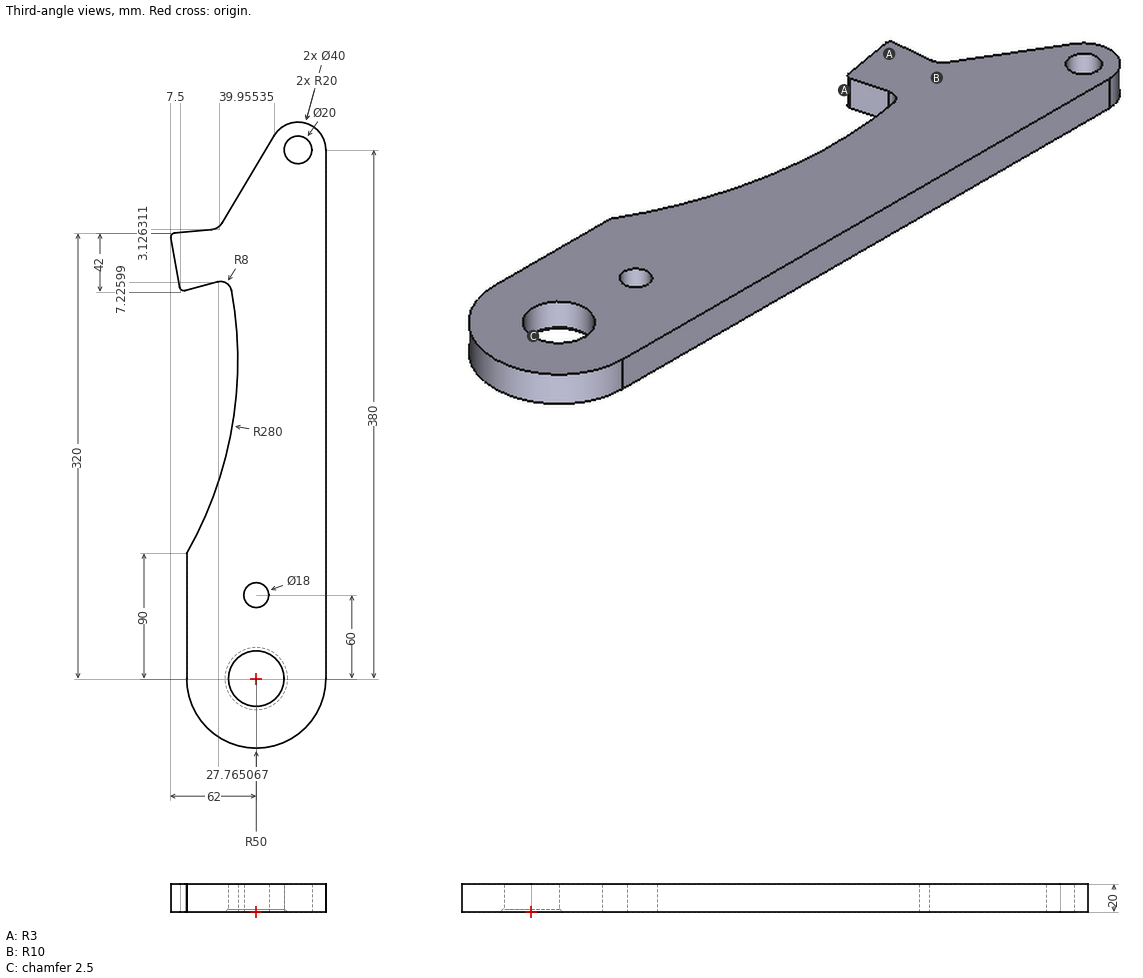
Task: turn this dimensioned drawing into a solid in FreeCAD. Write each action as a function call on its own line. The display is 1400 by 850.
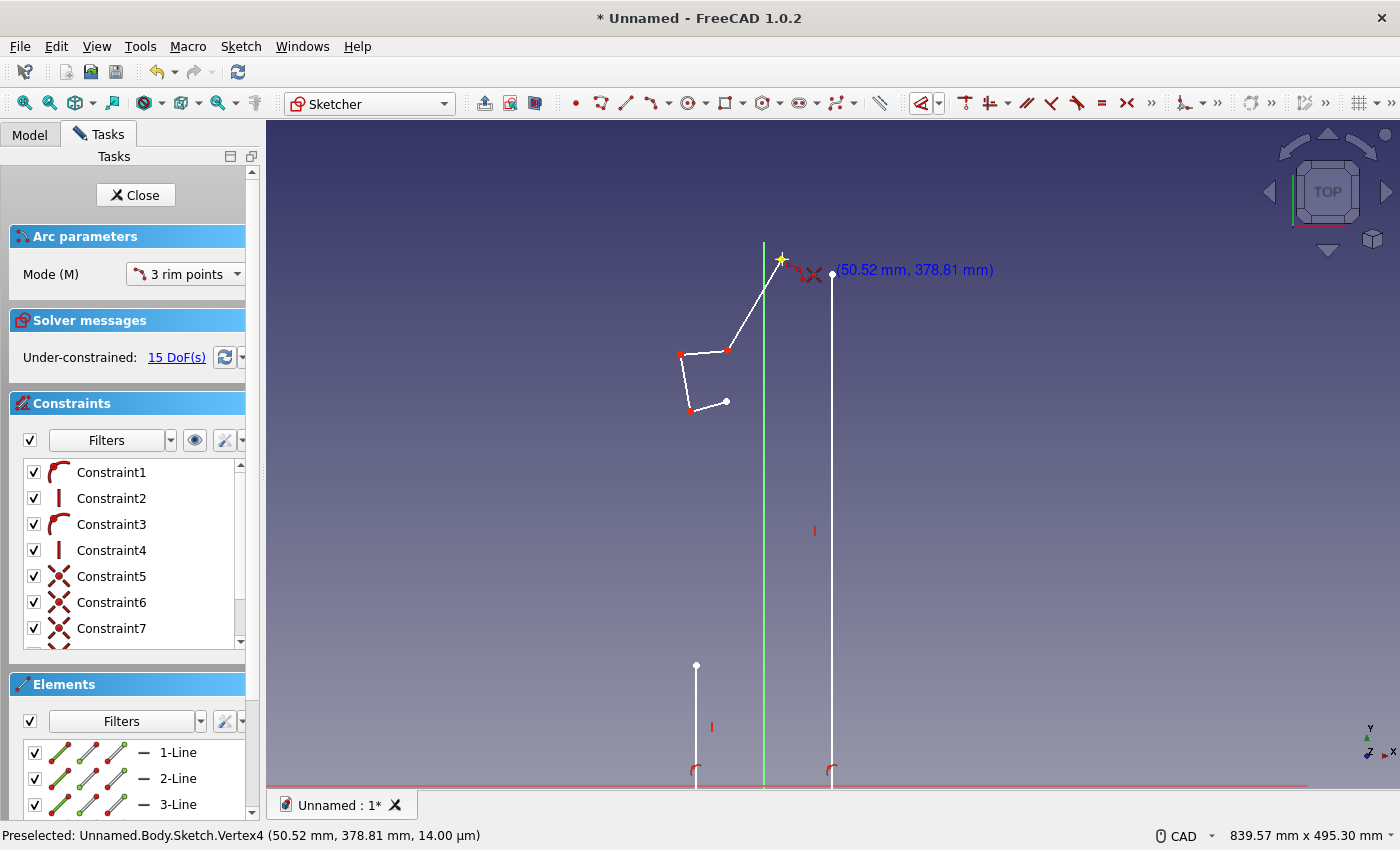
click(782, 260)
click(811, 247)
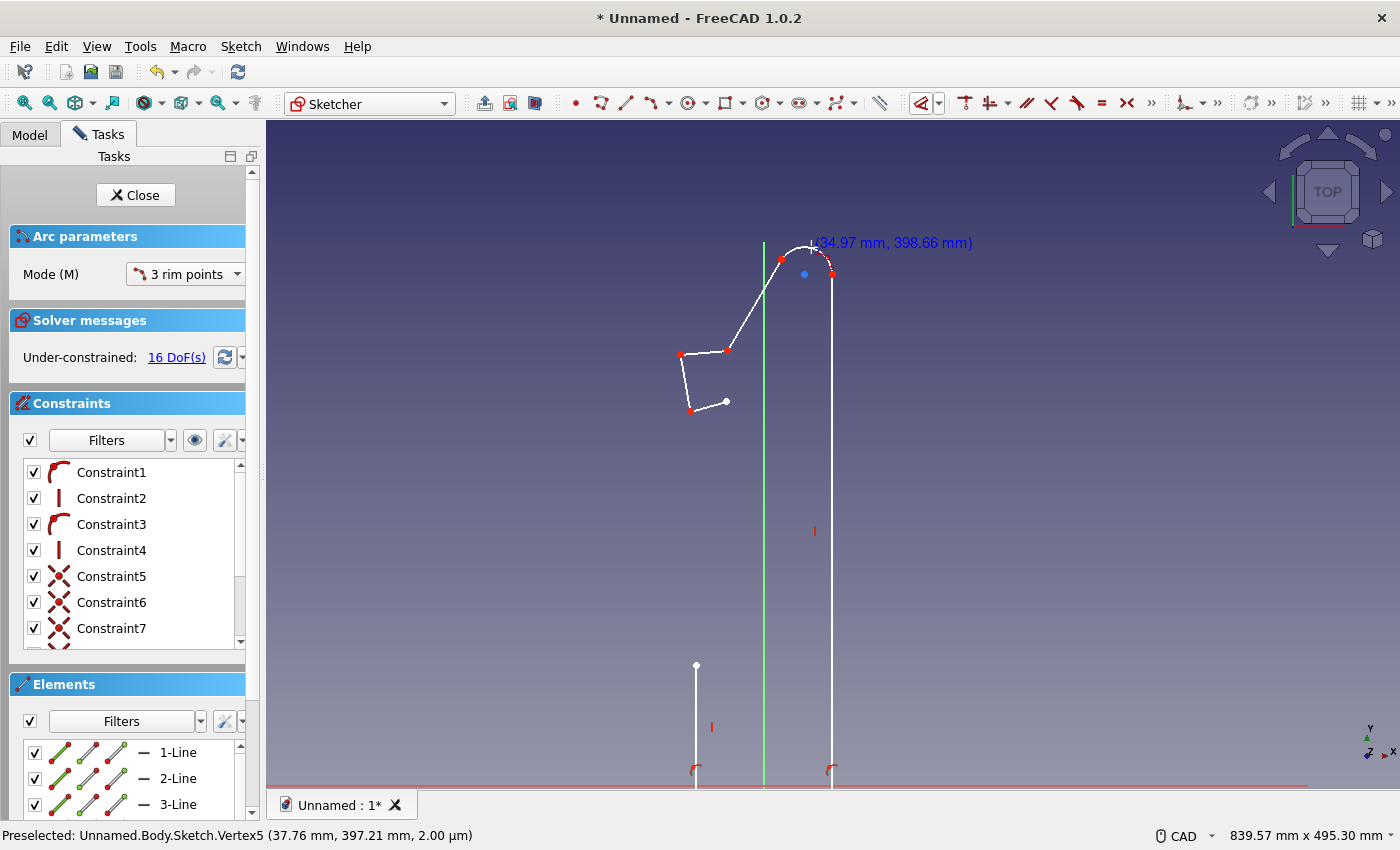
click(727, 402)
click(740, 410)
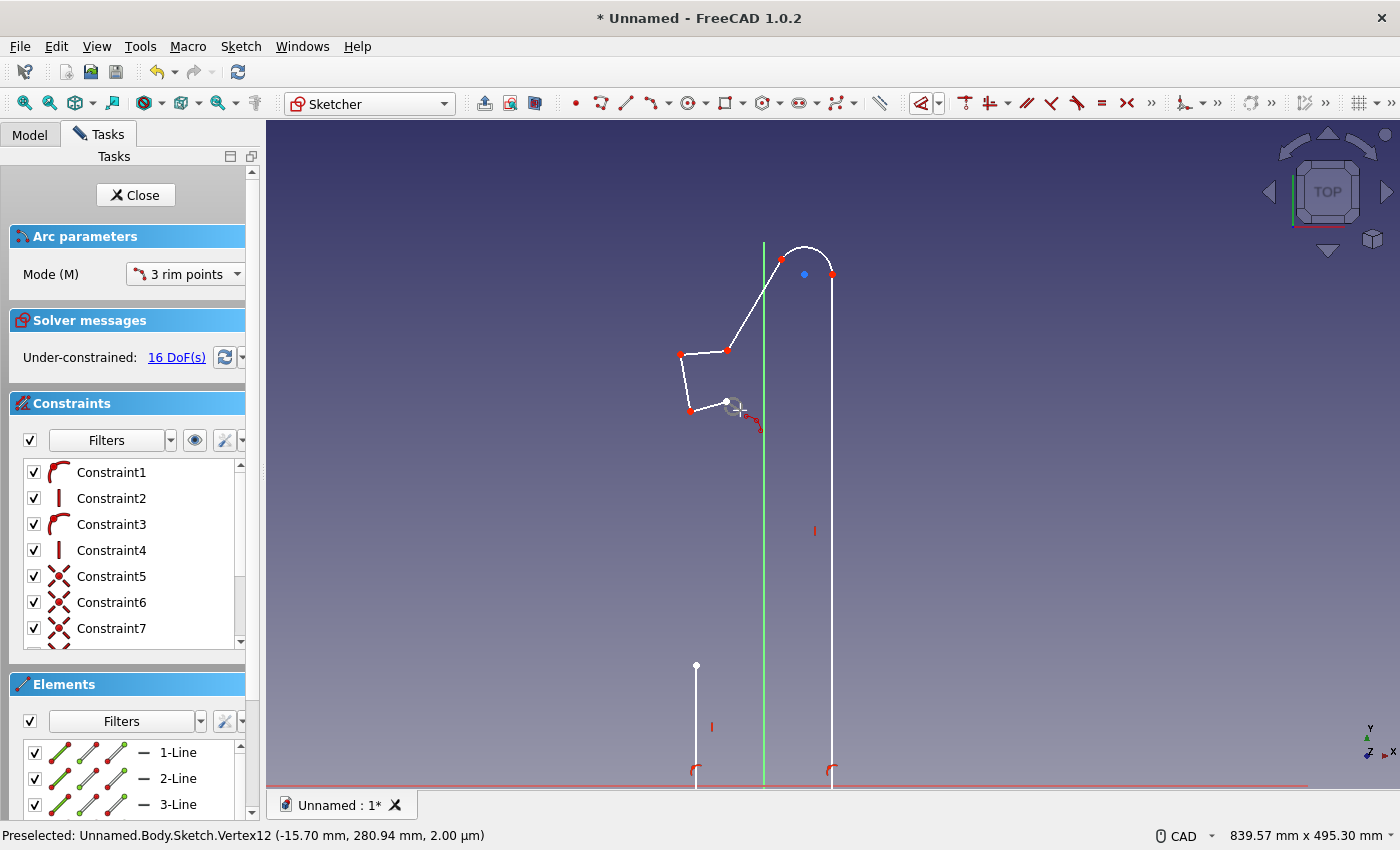
scroll(735, 403, up, 8)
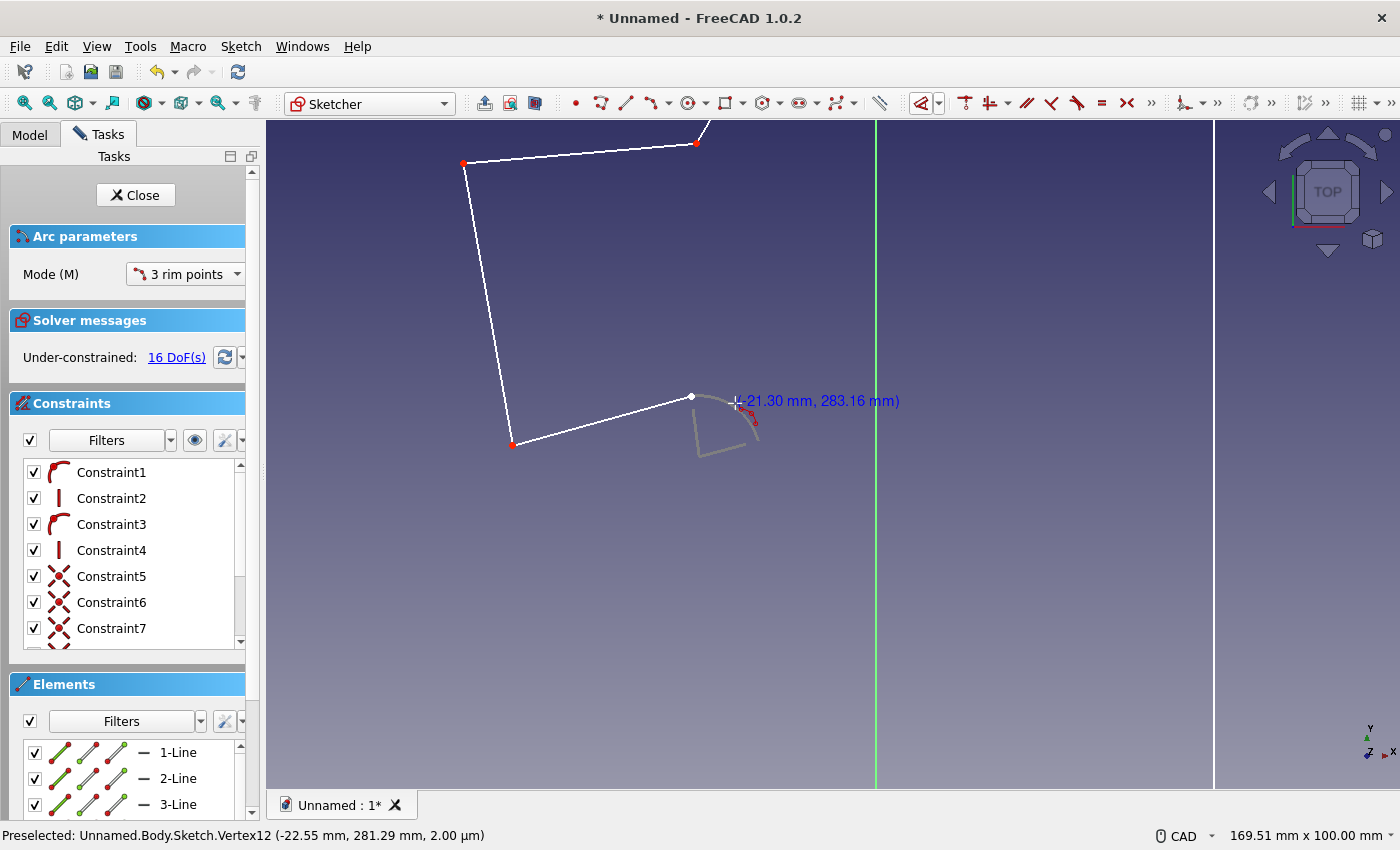
click(733, 399)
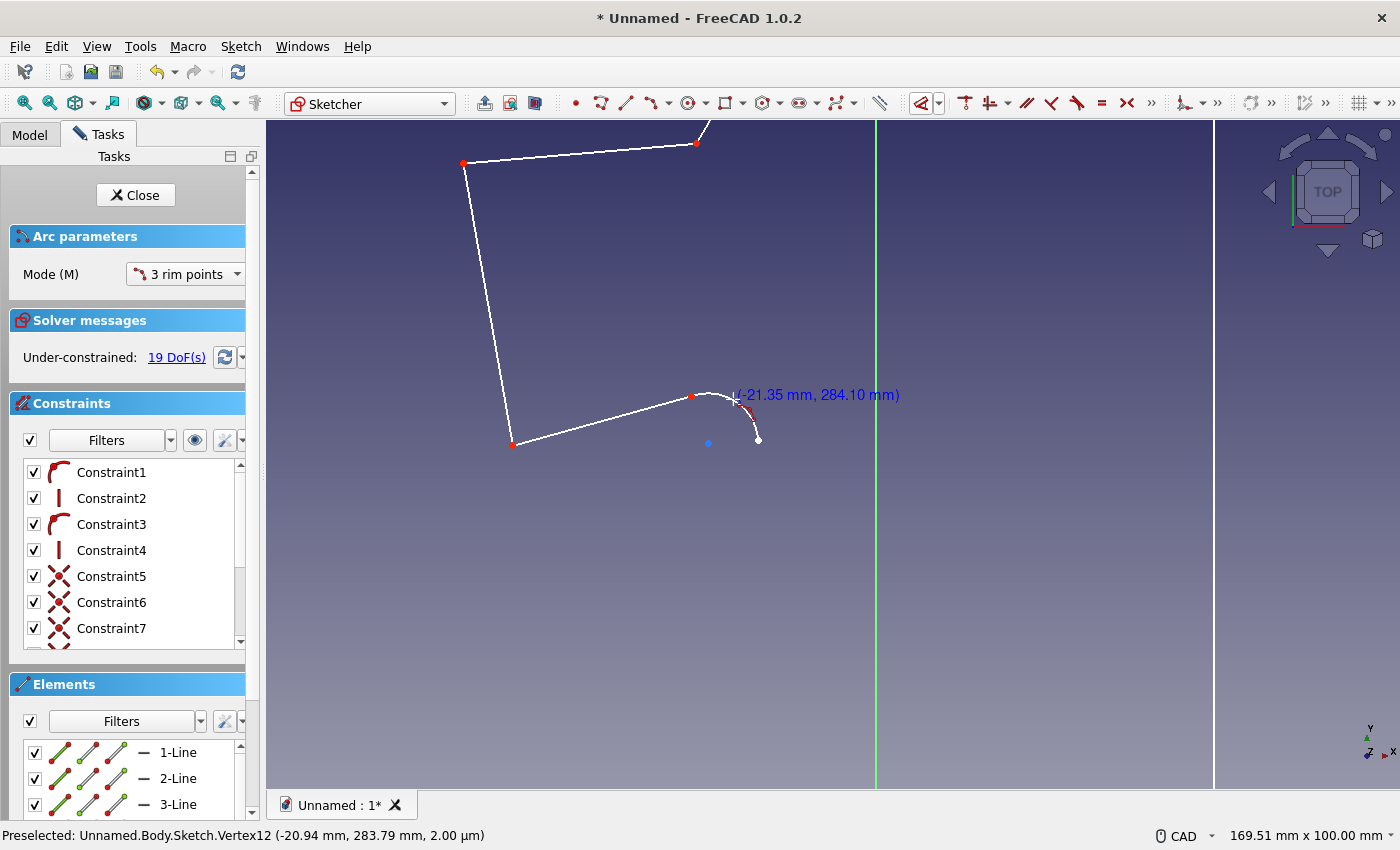
scroll(753, 348, down, 10)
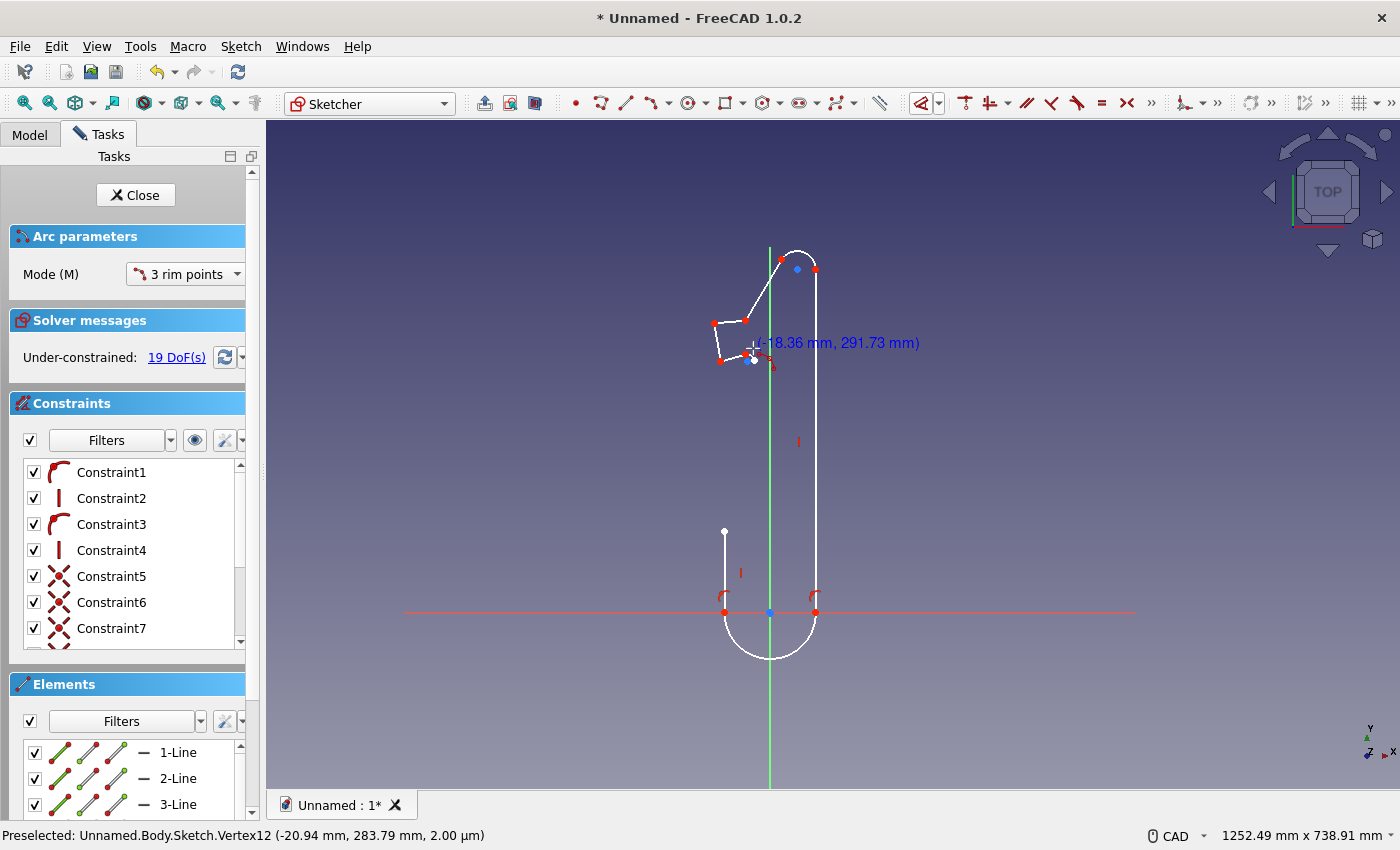
scroll(754, 360, up, 4)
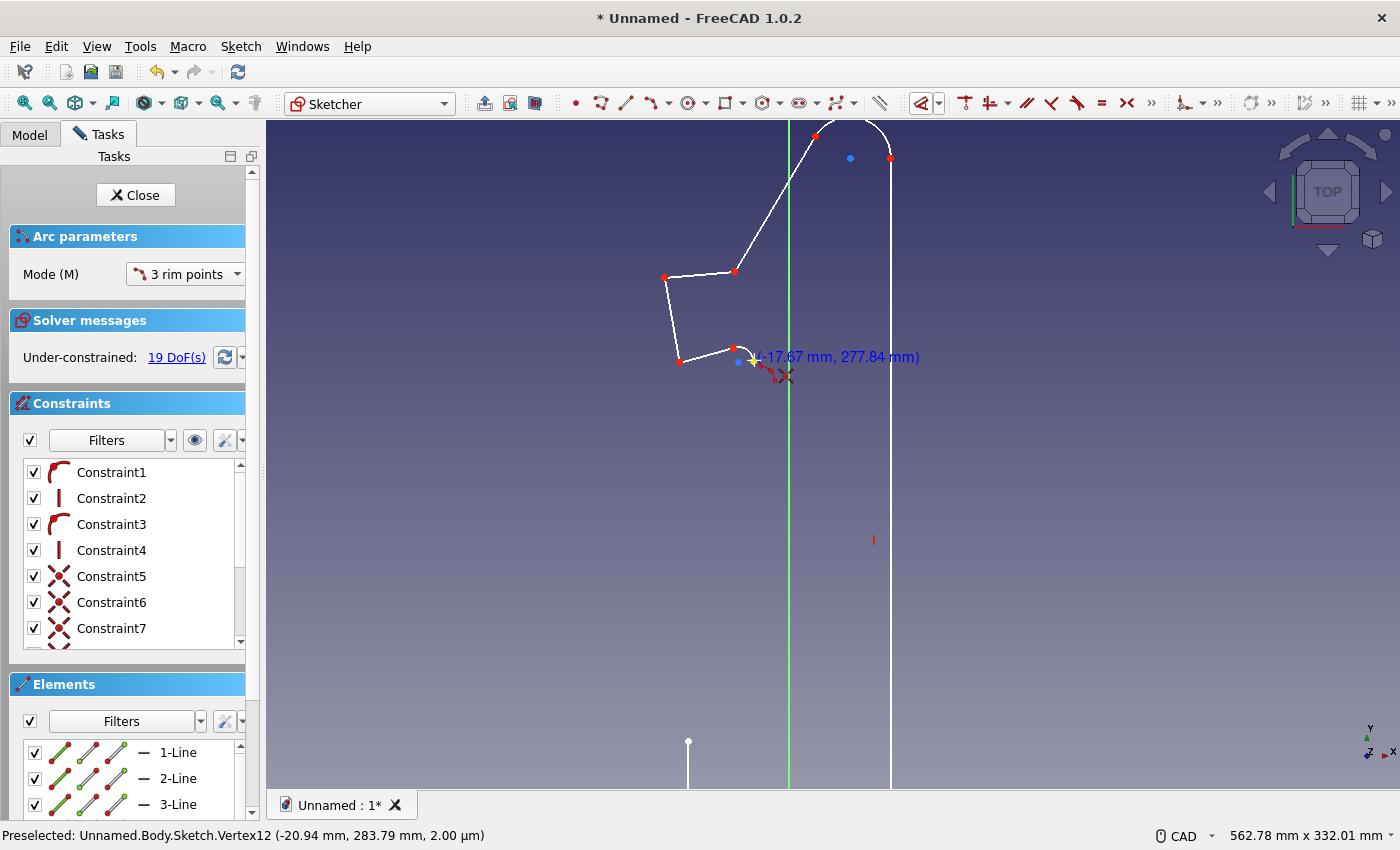
click(754, 362)
click(688, 741)
click(754, 556)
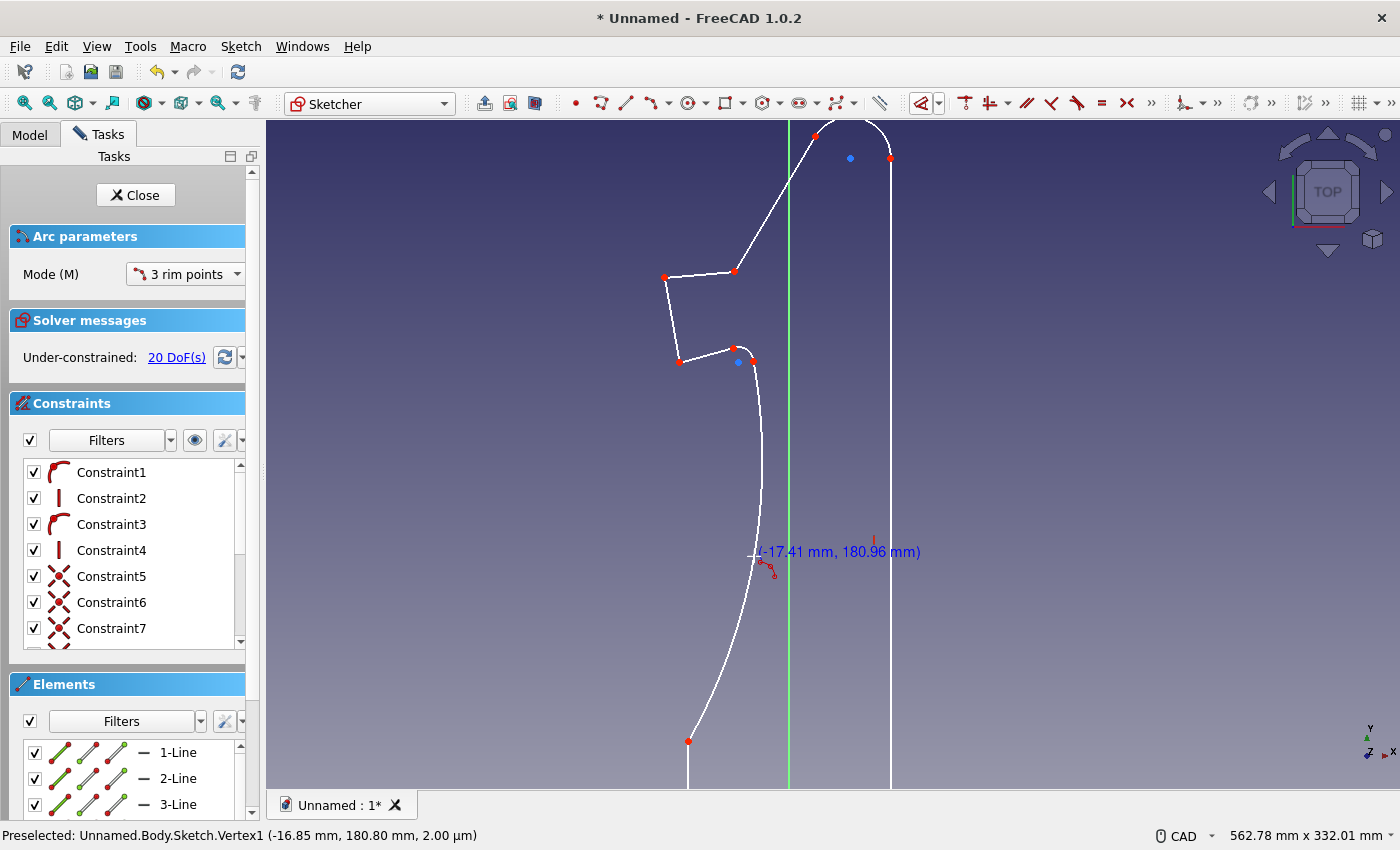
click(688, 104)